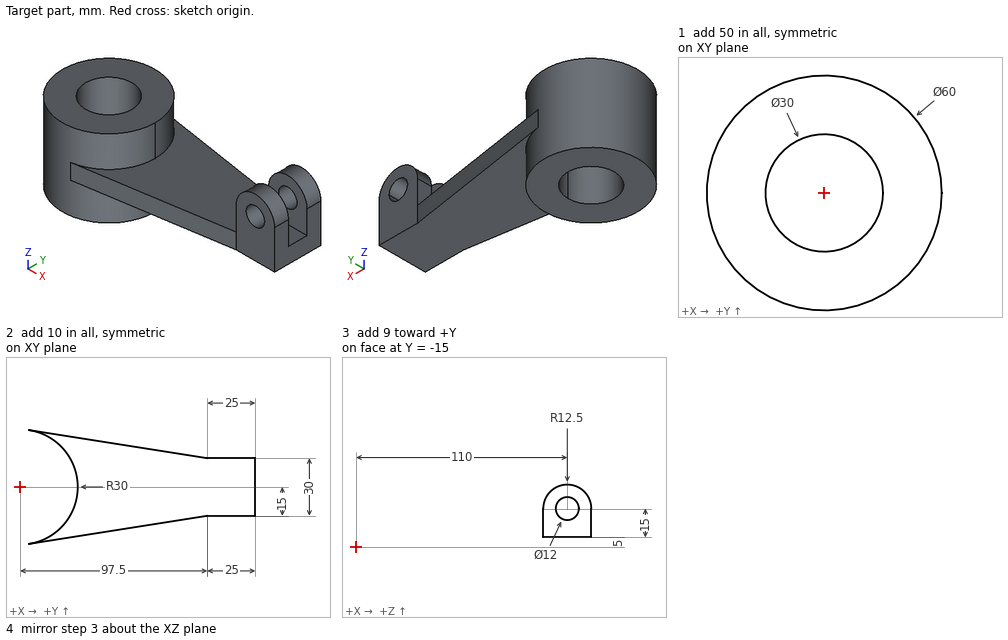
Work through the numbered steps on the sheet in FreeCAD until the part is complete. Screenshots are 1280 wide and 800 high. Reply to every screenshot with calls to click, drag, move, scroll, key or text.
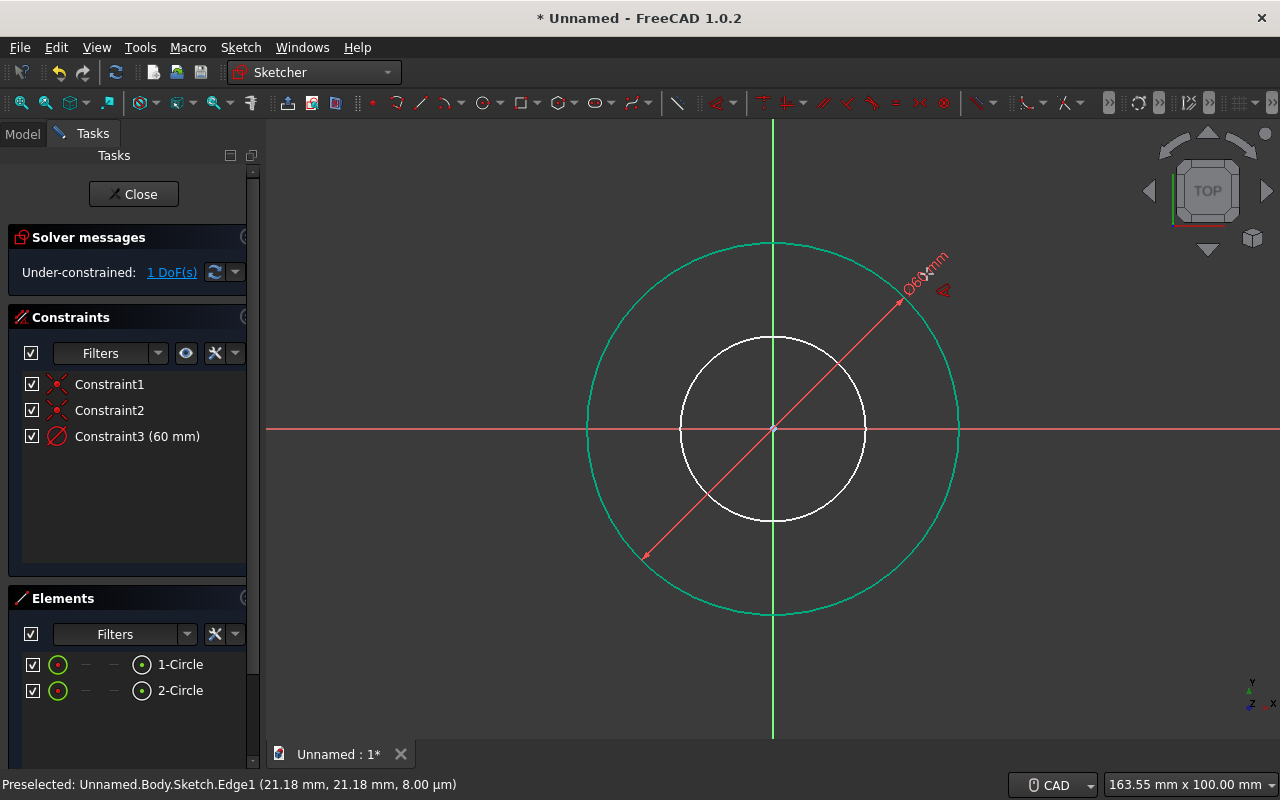
click(838, 363)
click(860, 340)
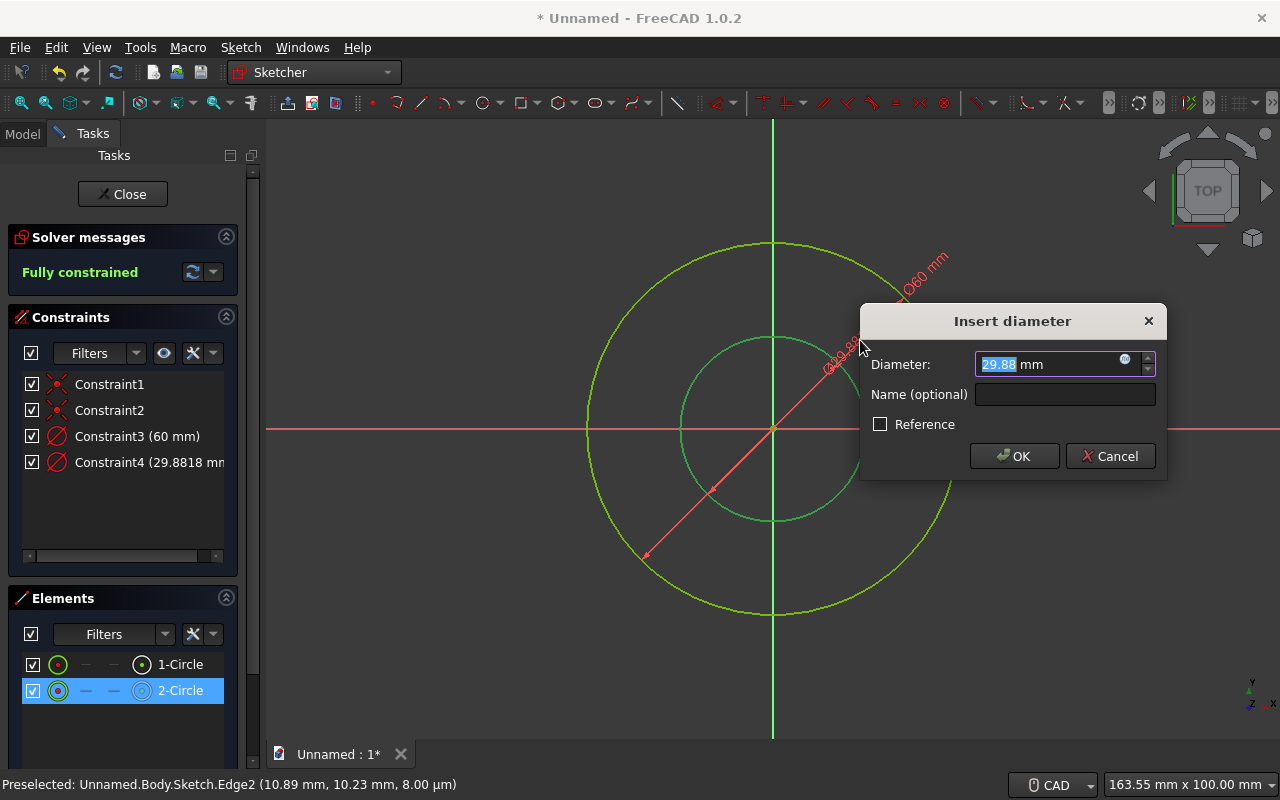
text(30)
key(Return)
key(Escape)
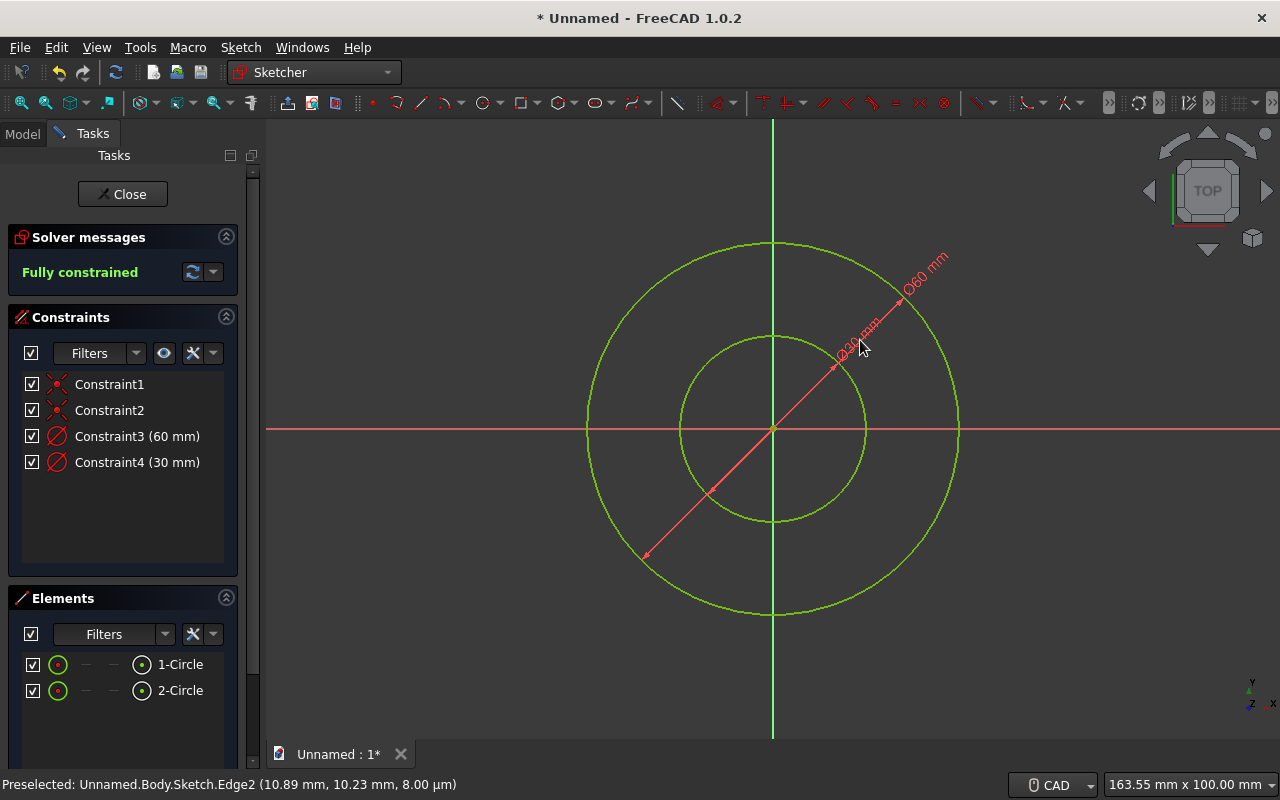
click(123, 194)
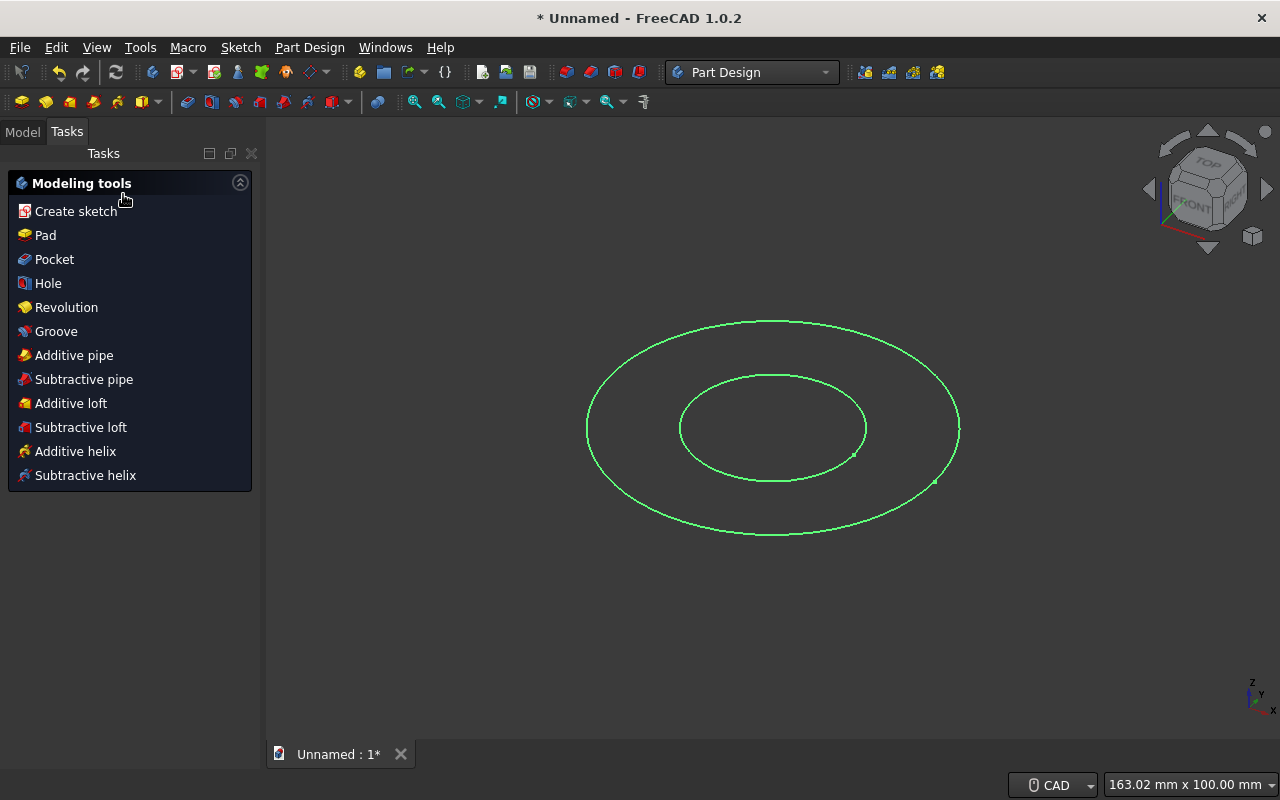
click(22, 102)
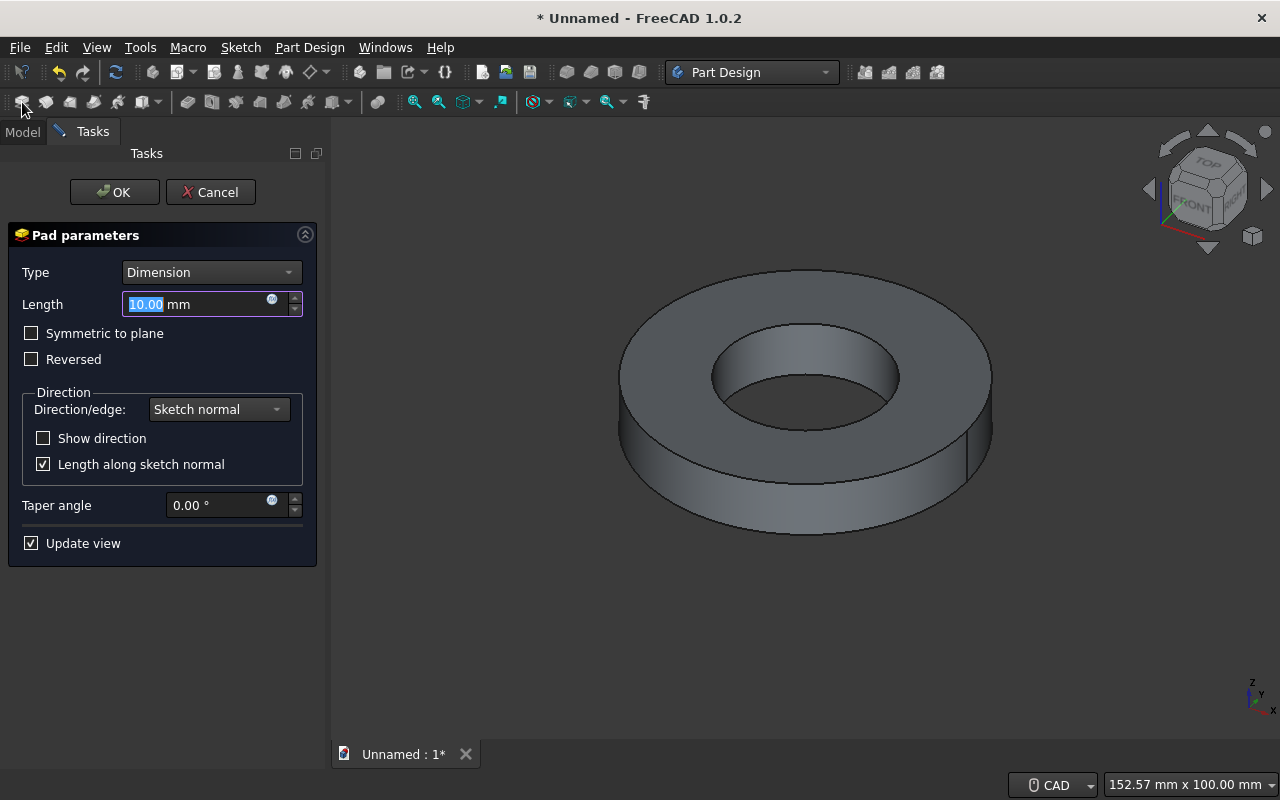
text(50)
key(Tab)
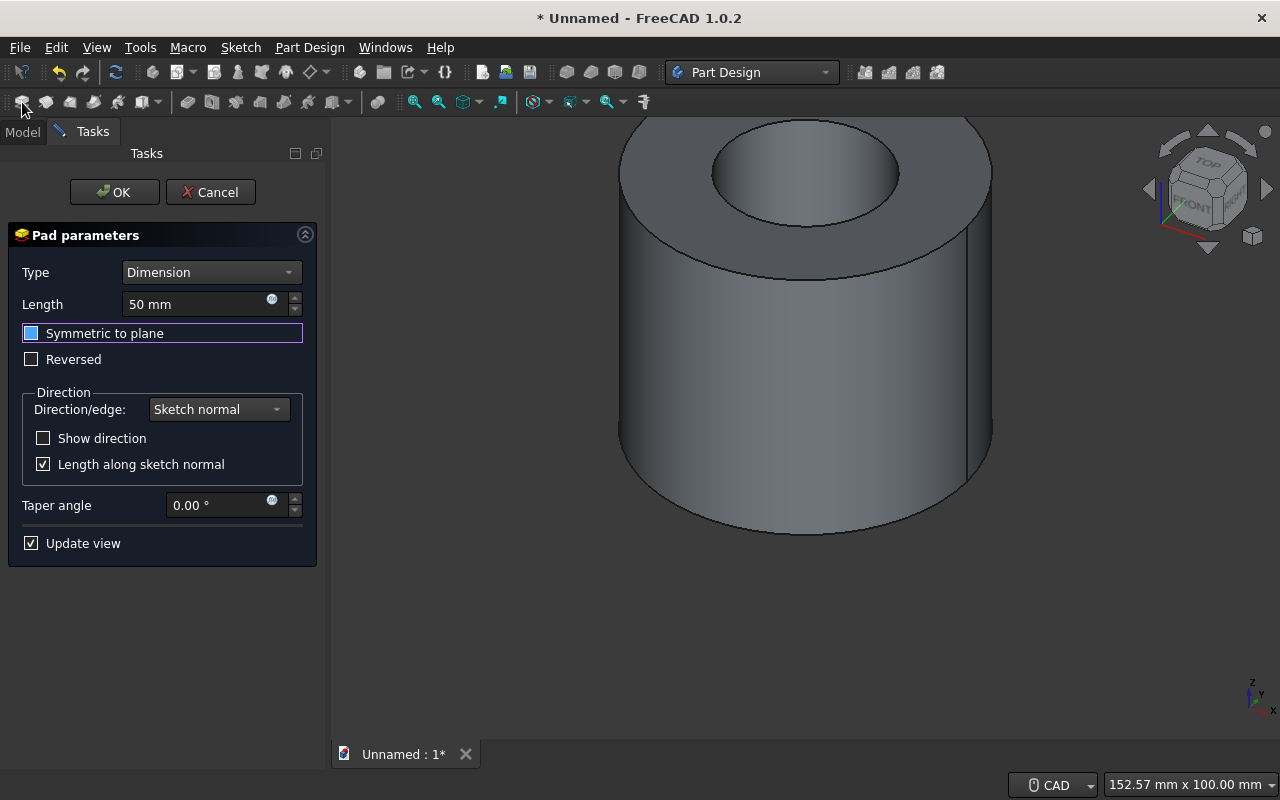
click(30, 333)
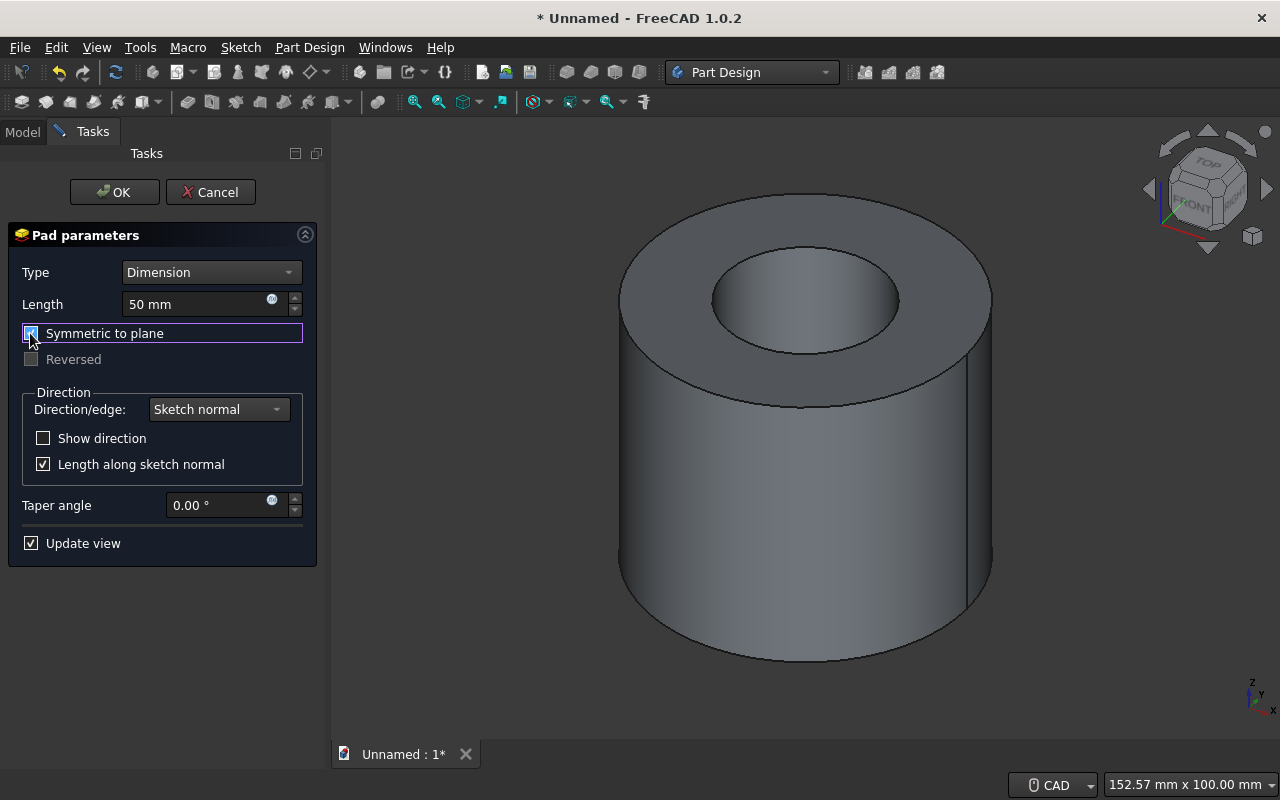
click(115, 192)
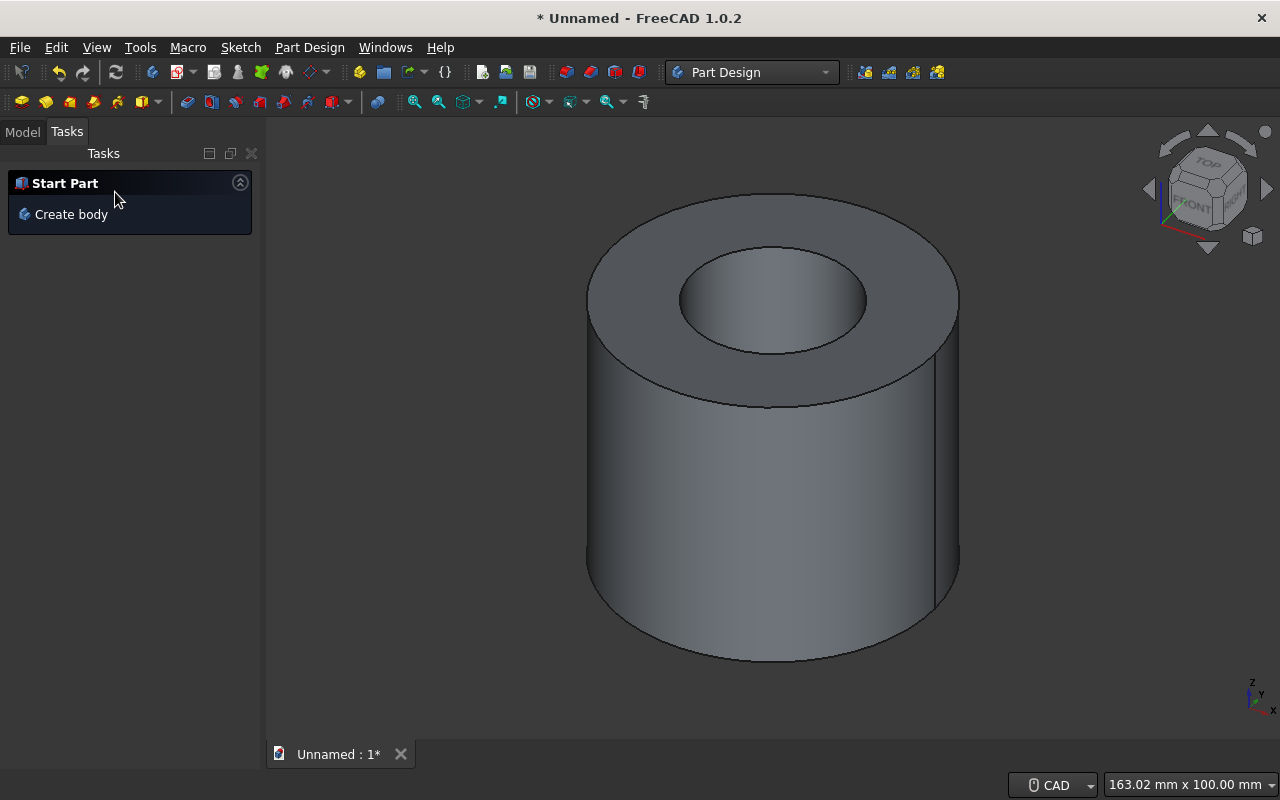
click(178, 72)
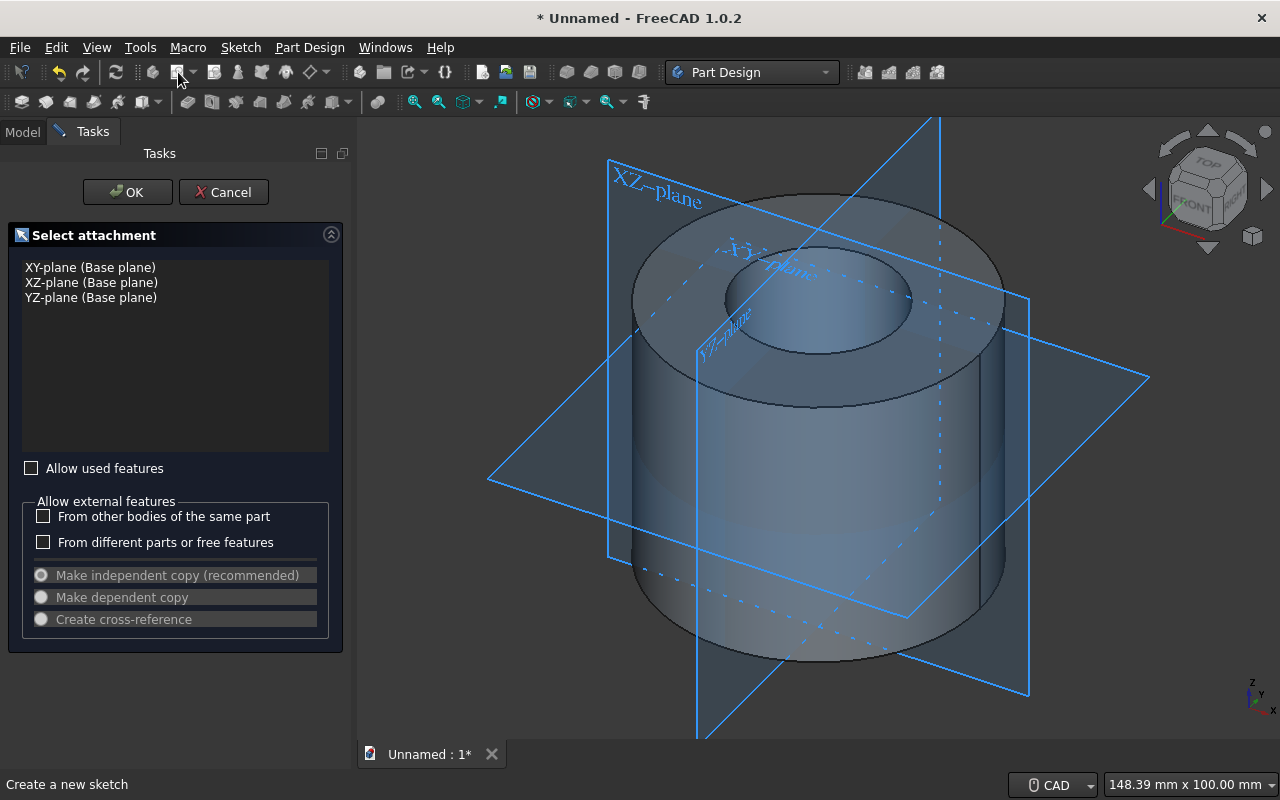
click(82, 268)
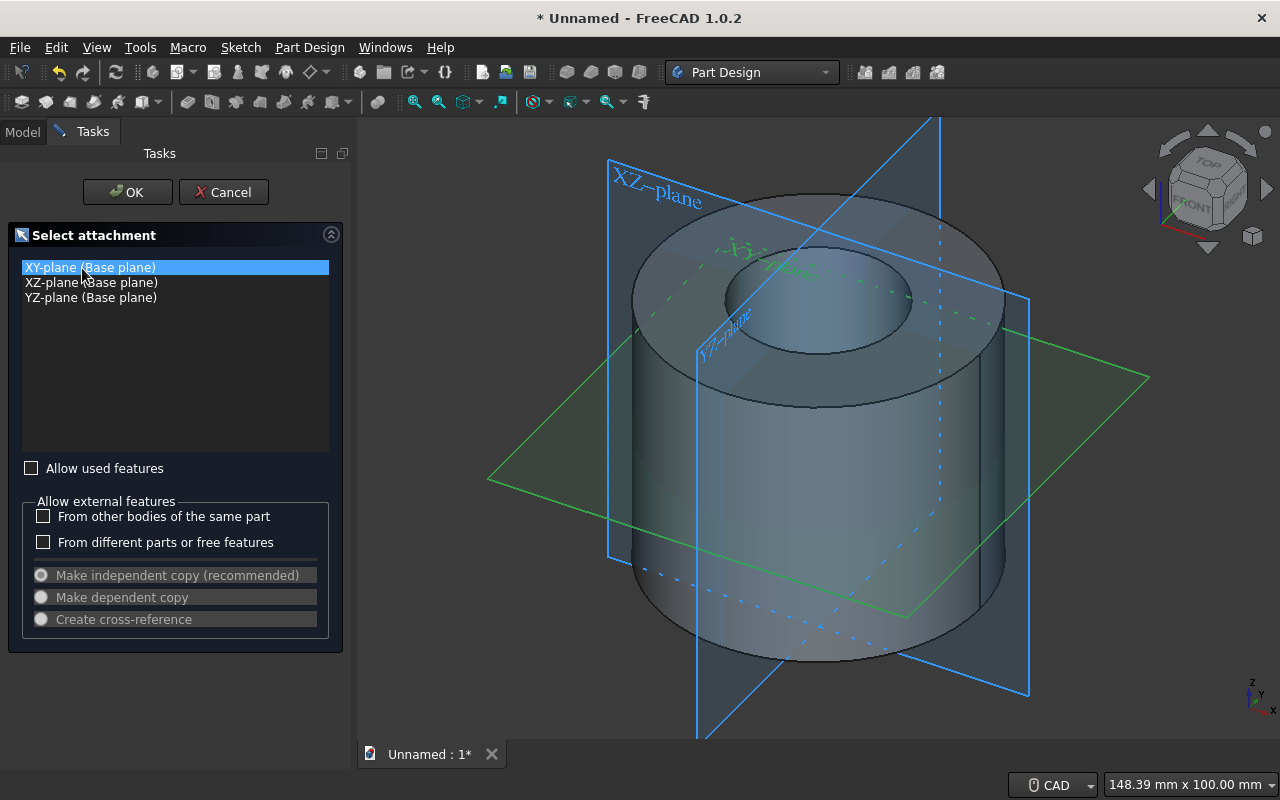
click(128, 192)